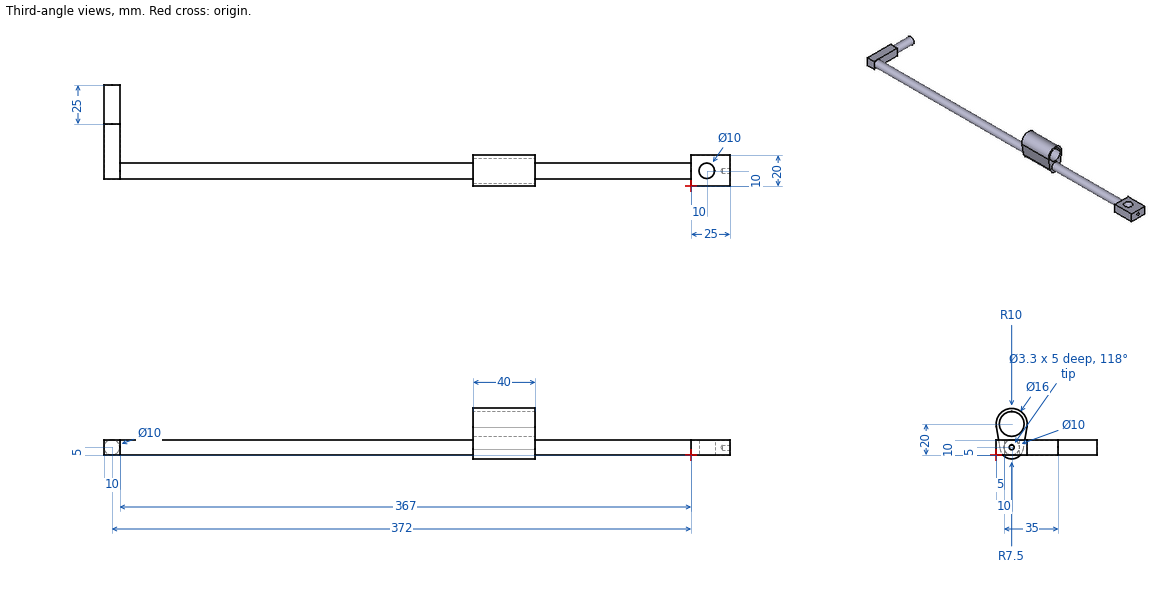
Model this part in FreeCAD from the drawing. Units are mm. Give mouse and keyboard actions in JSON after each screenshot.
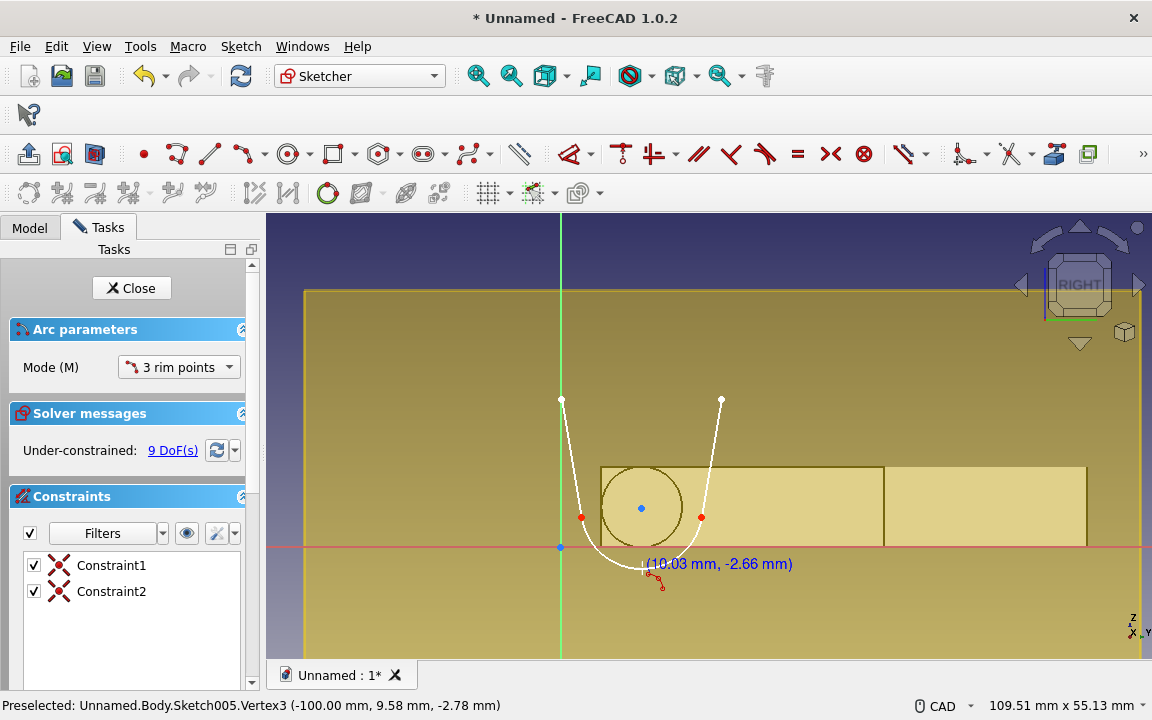
{"action": "scroll", "coordinate": [562, 399], "scroll_direction": "up", "scroll_amount": 14}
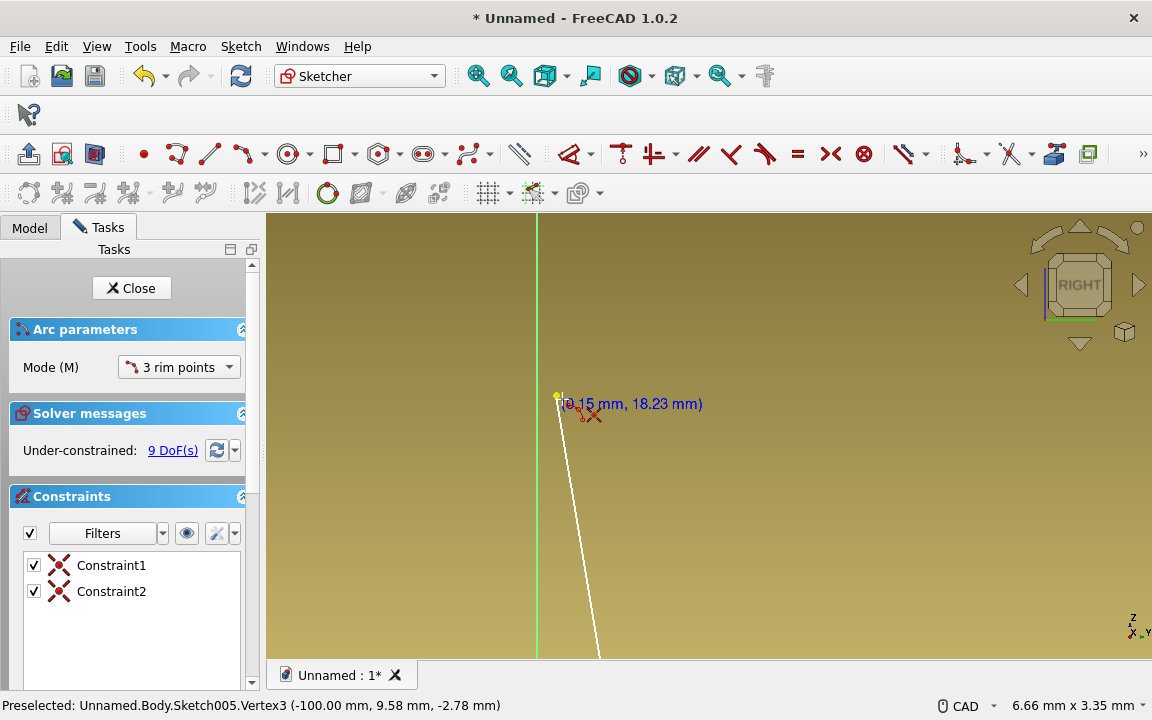
{"action": "left_click", "coordinate": [556, 396]}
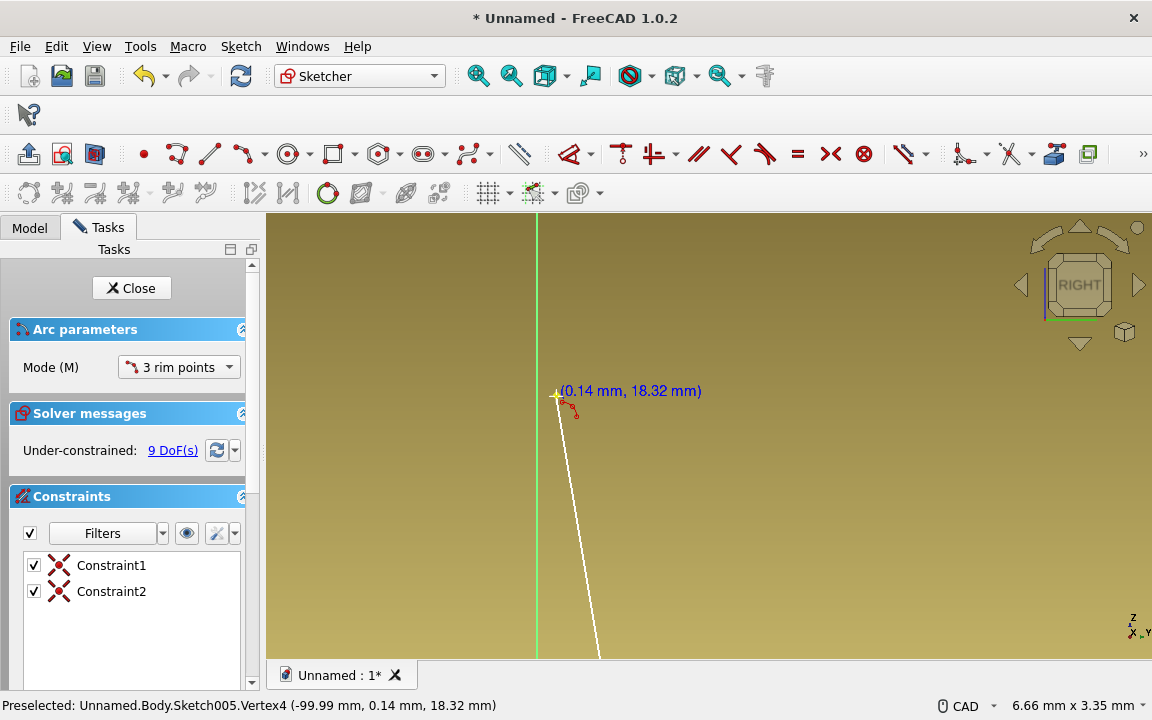
{"action": "scroll", "coordinate": [562, 399], "scroll_direction": "down", "scroll_amount": 14}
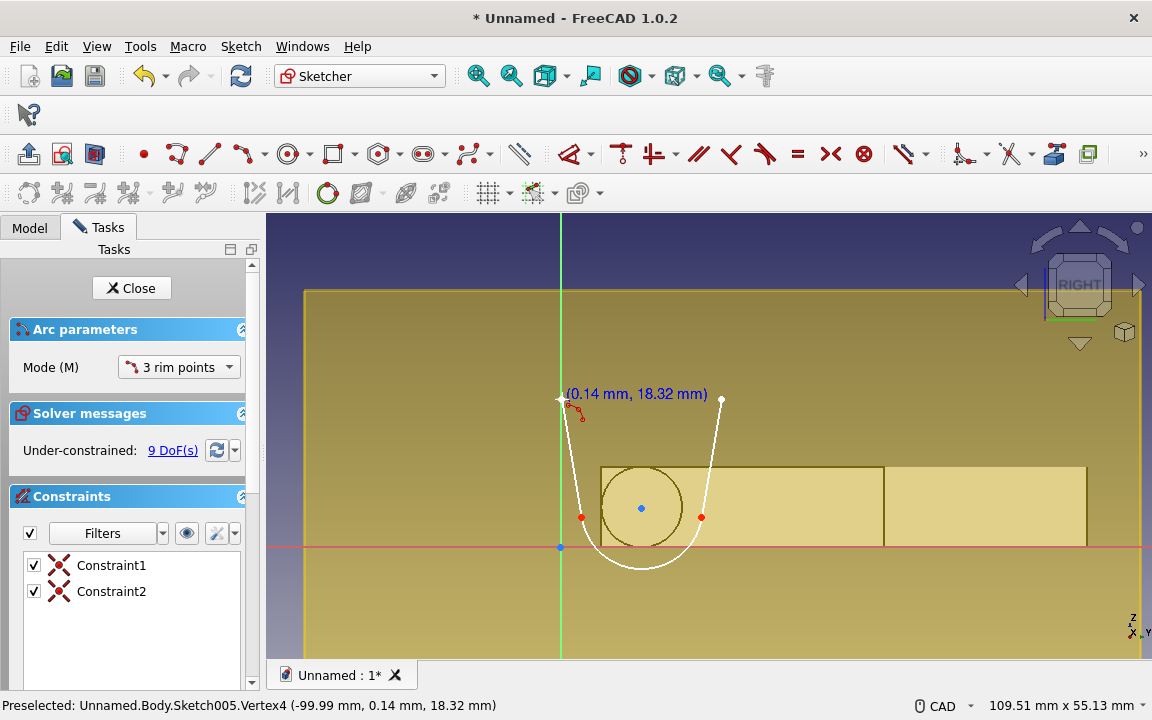
{"action": "left_click", "coordinate": [722, 400]}
{"action": "left_click", "coordinate": [642, 305]}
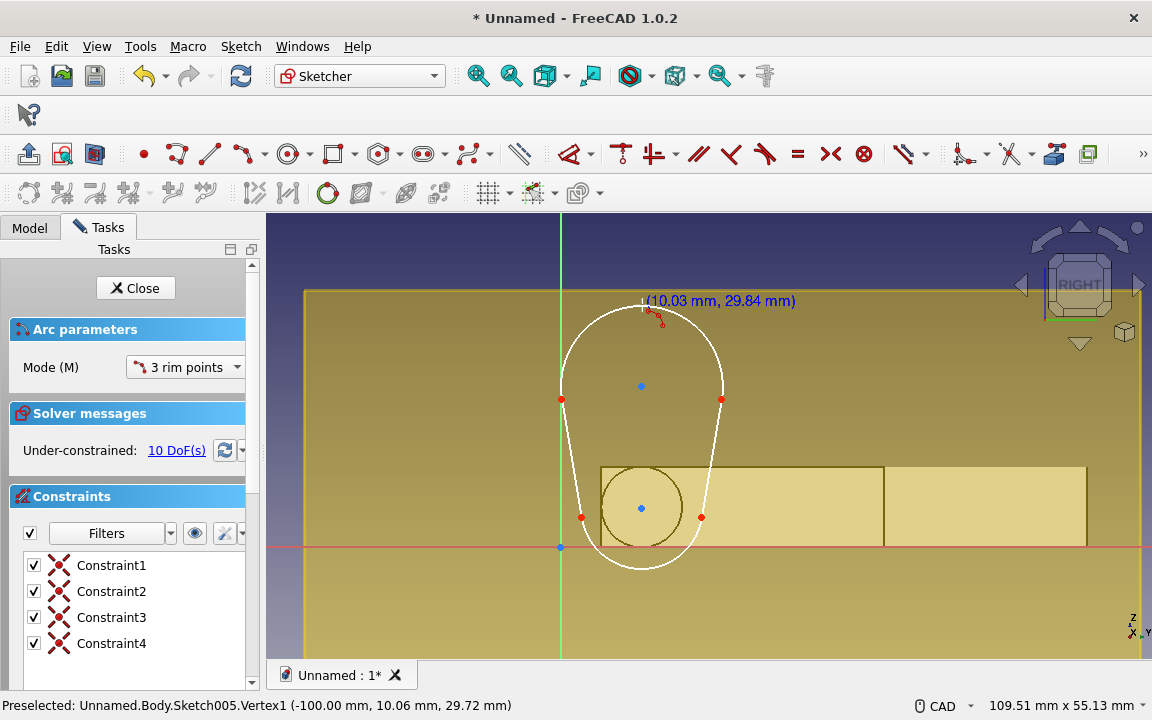
{"action": "key", "text": "g c"}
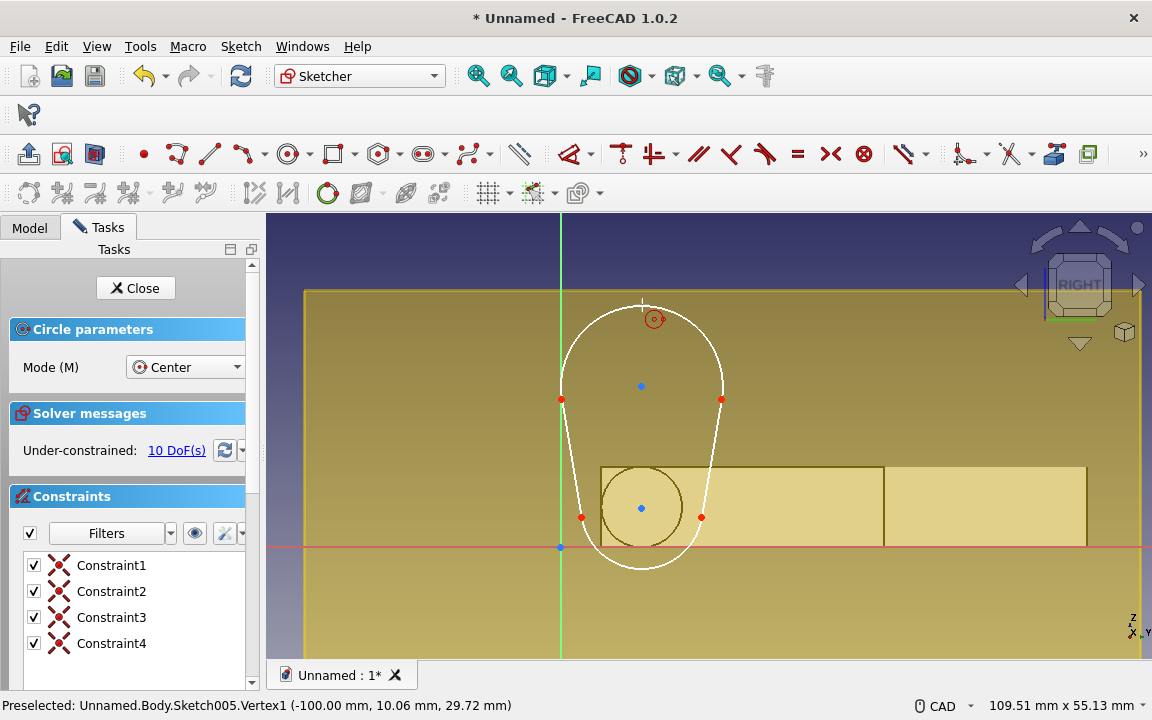
{"action": "left_click", "coordinate": [642, 386]}
{"action": "mouse_move", "coordinate": [687, 340]}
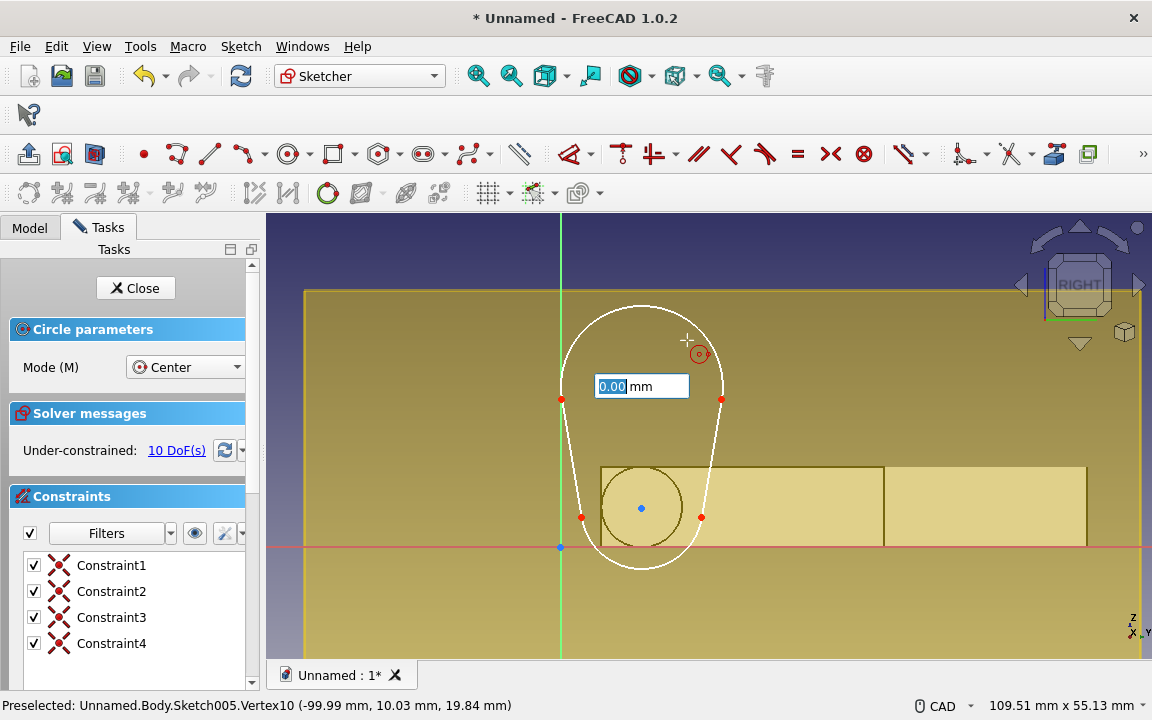
{"action": "type", "text": "16"}
{"action": "key", "text": "Return"}
{"action": "key", "text": "Escape"}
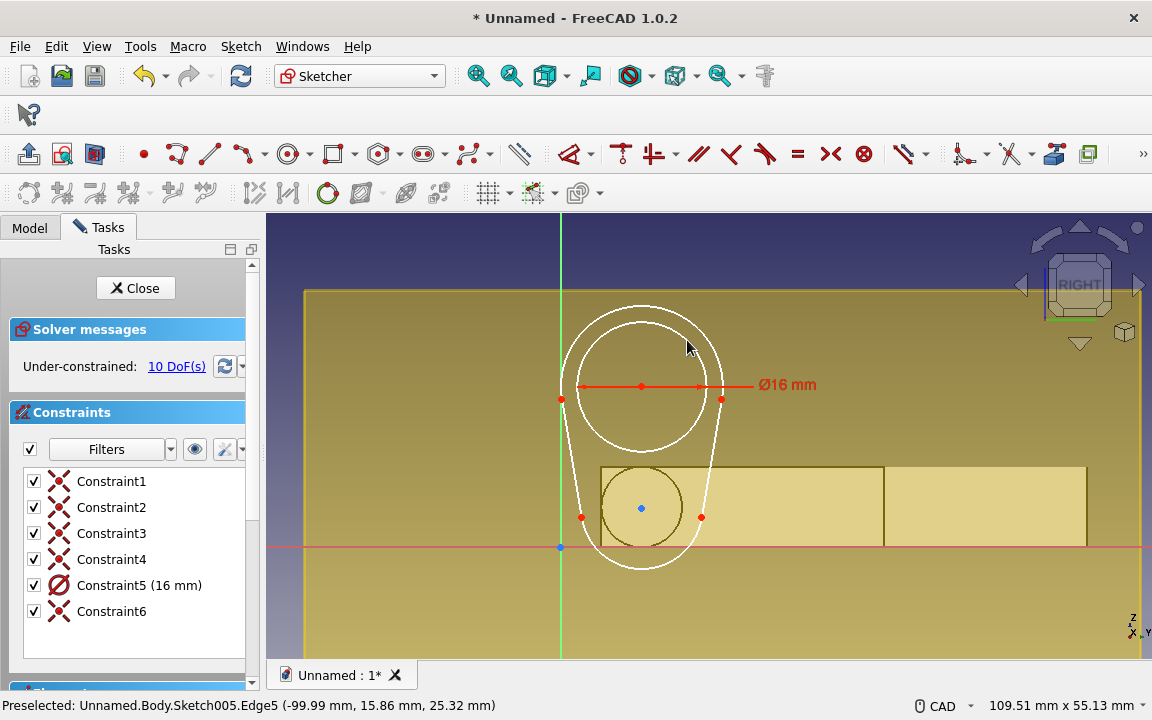
{"action": "left_click", "coordinate": [716, 435]}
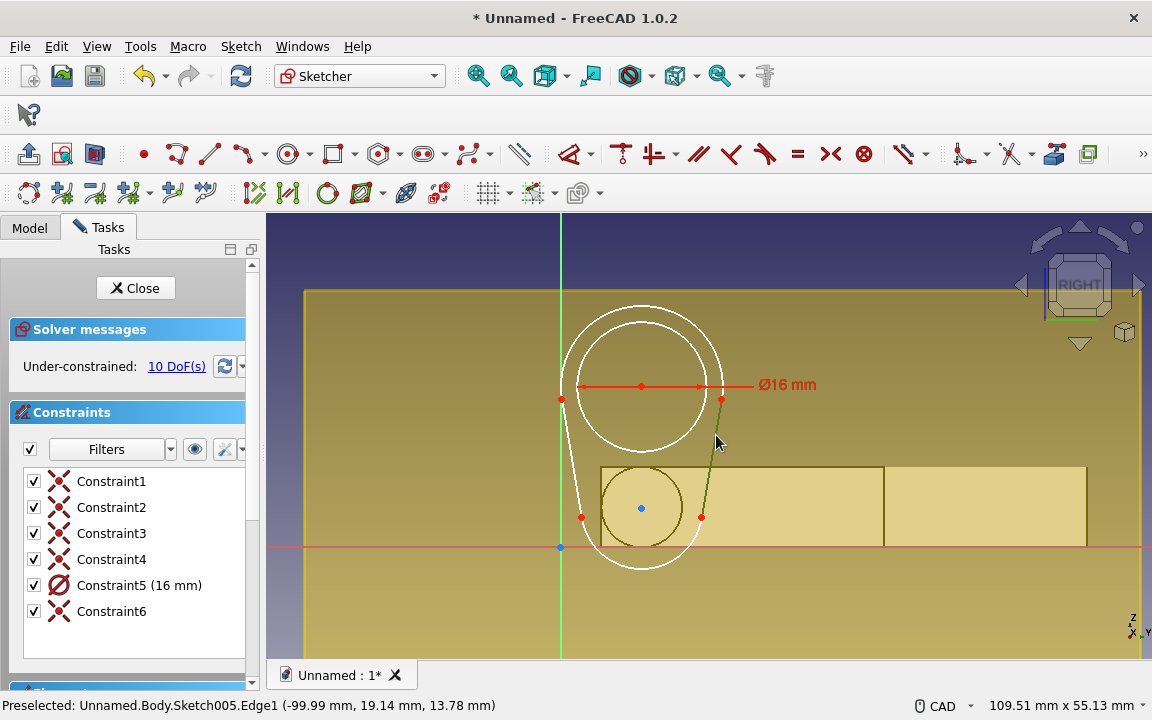
{"action": "left_click", "coordinate": [609, 560]}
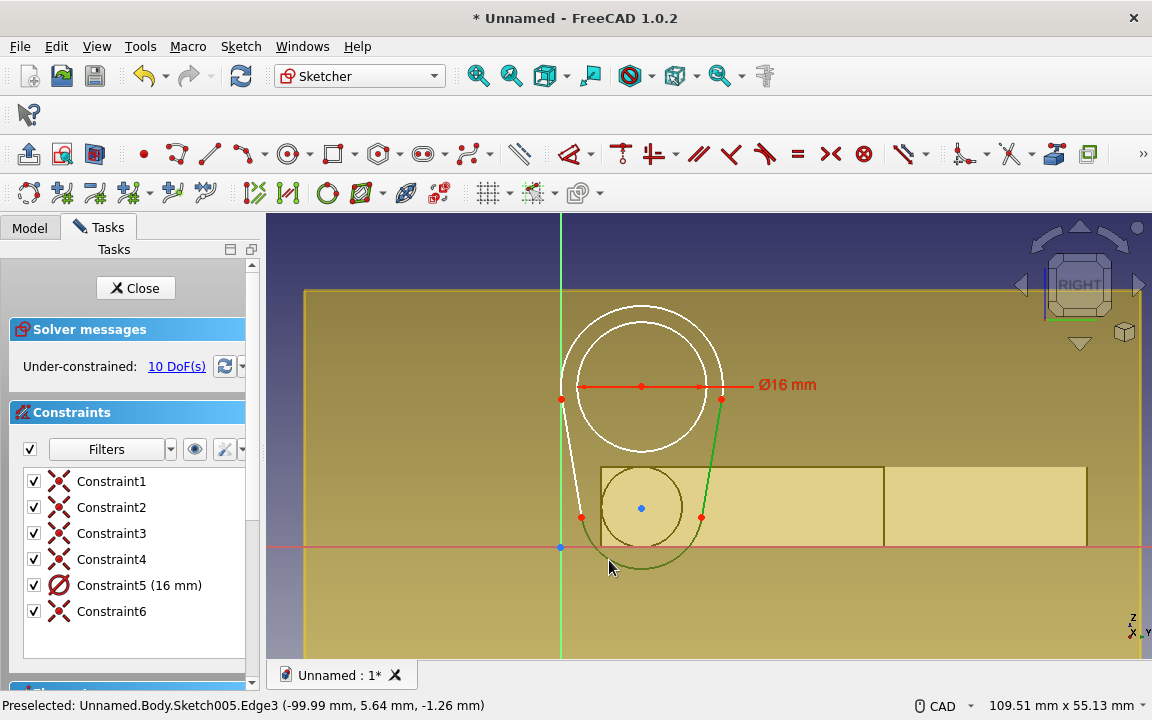
{"action": "key", "text": "t"}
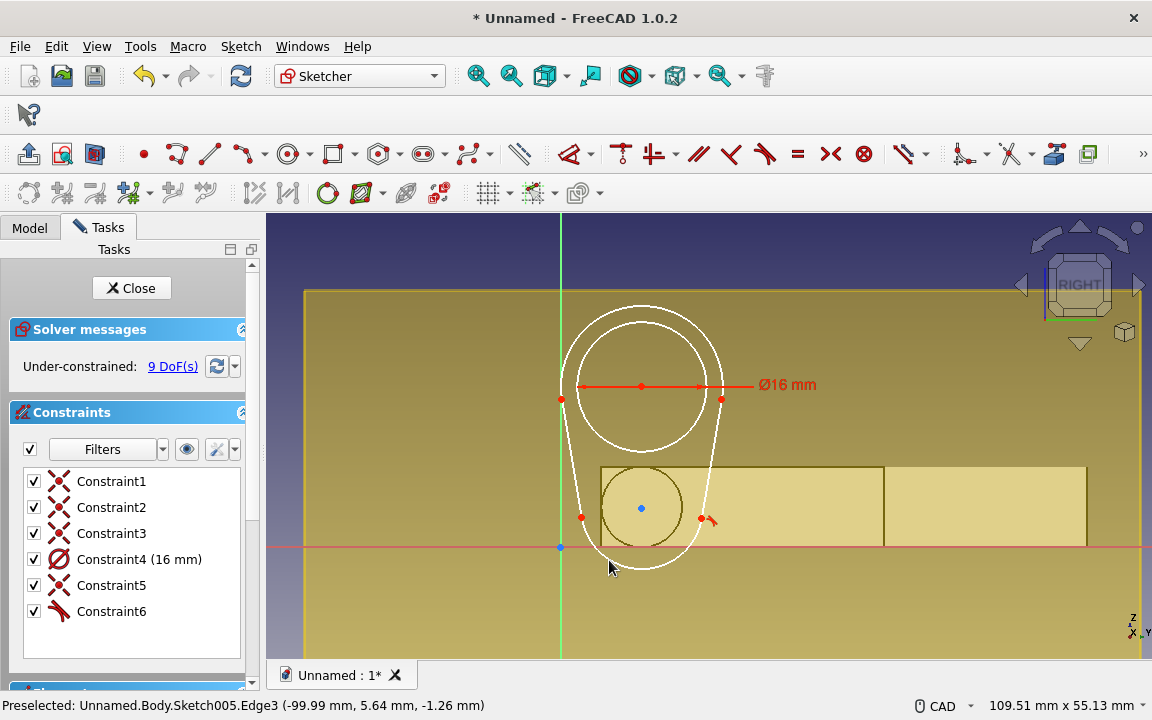
{"action": "left_click", "coordinate": [716, 435]}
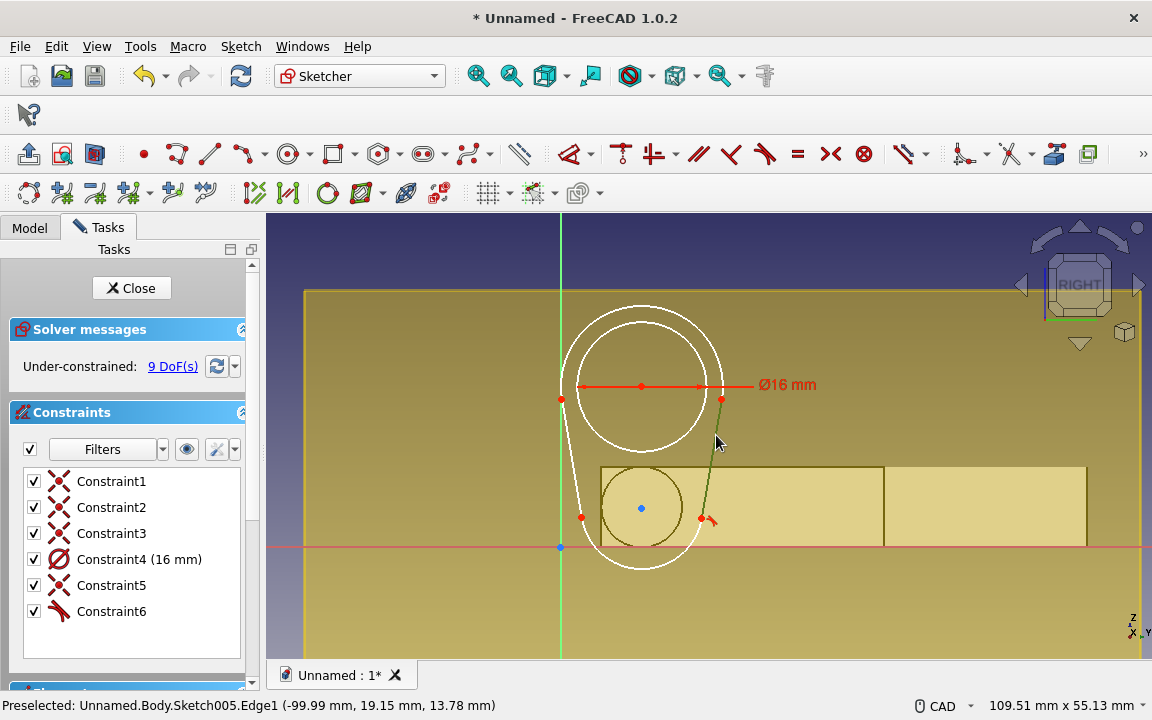
{"action": "left_click", "coordinate": [694, 325]}